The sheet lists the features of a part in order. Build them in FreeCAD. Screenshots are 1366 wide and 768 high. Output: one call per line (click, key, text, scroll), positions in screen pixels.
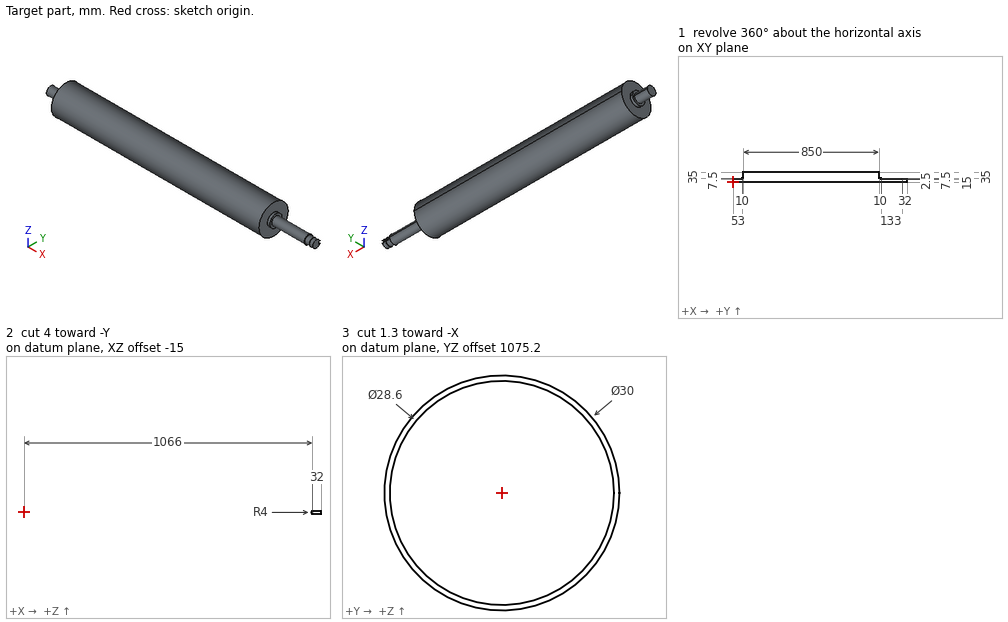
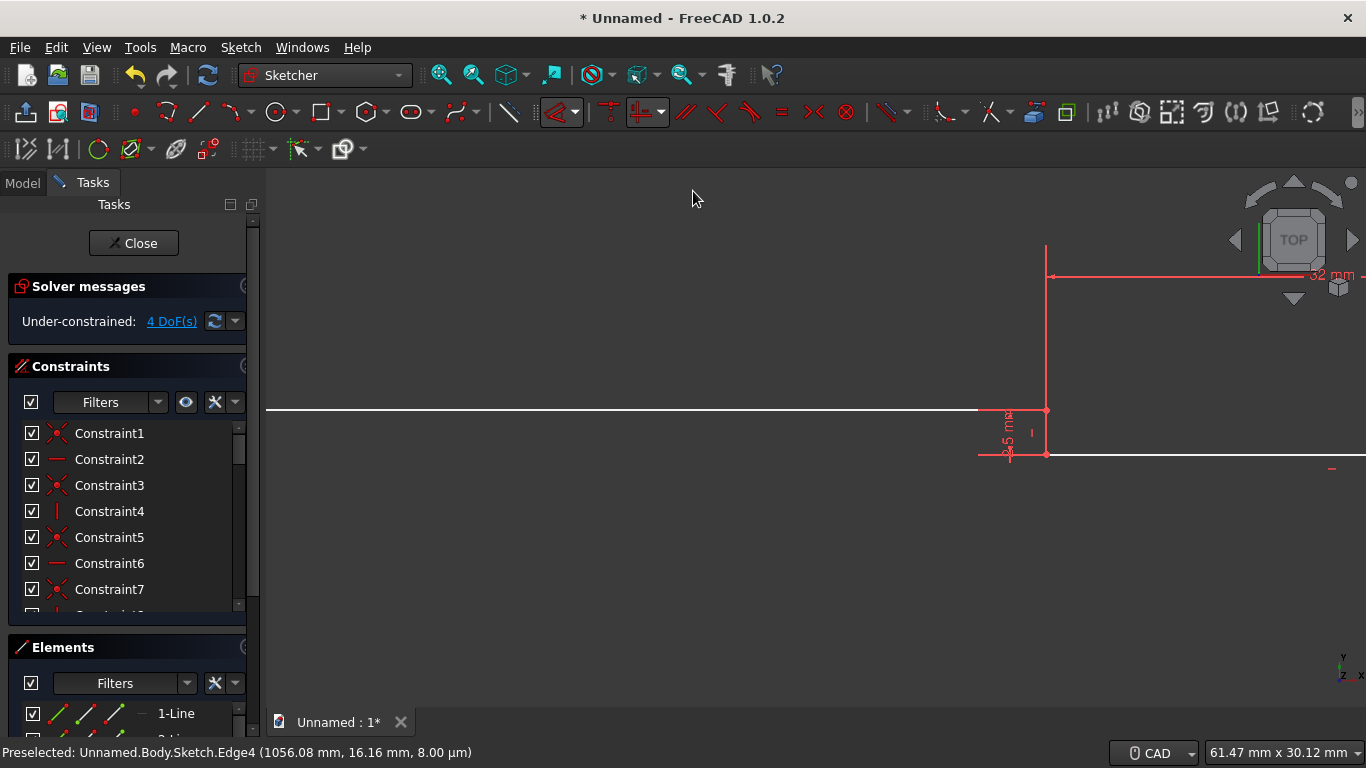
scroll(1124, 448, down, 16)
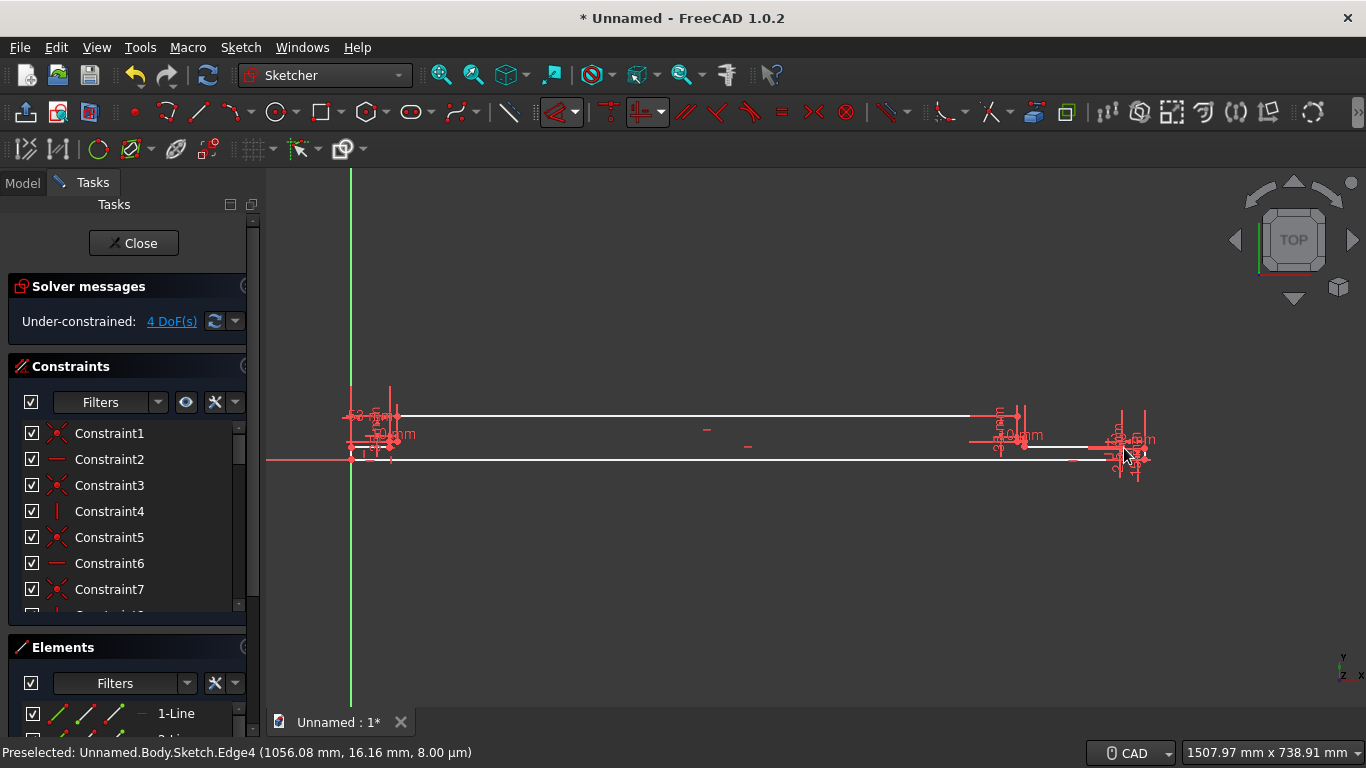
click(1092, 447)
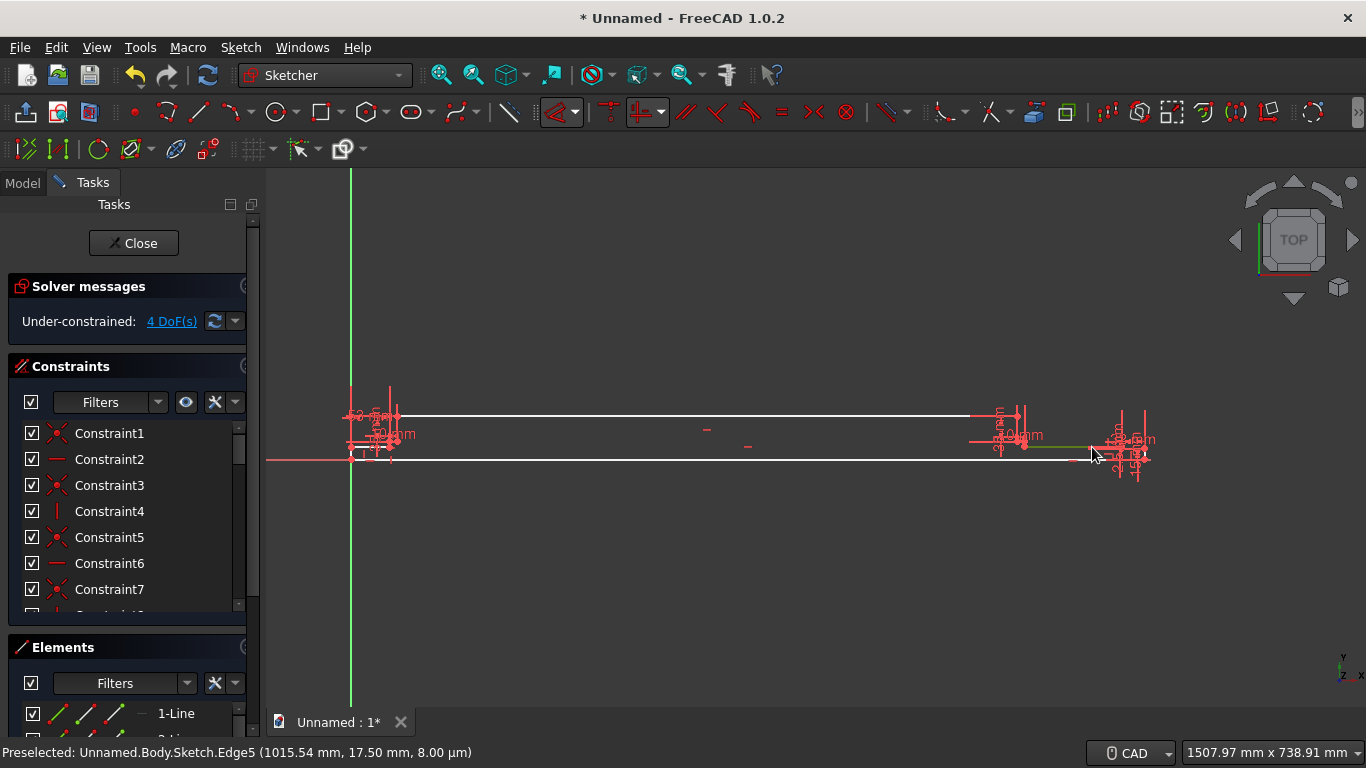
key(l)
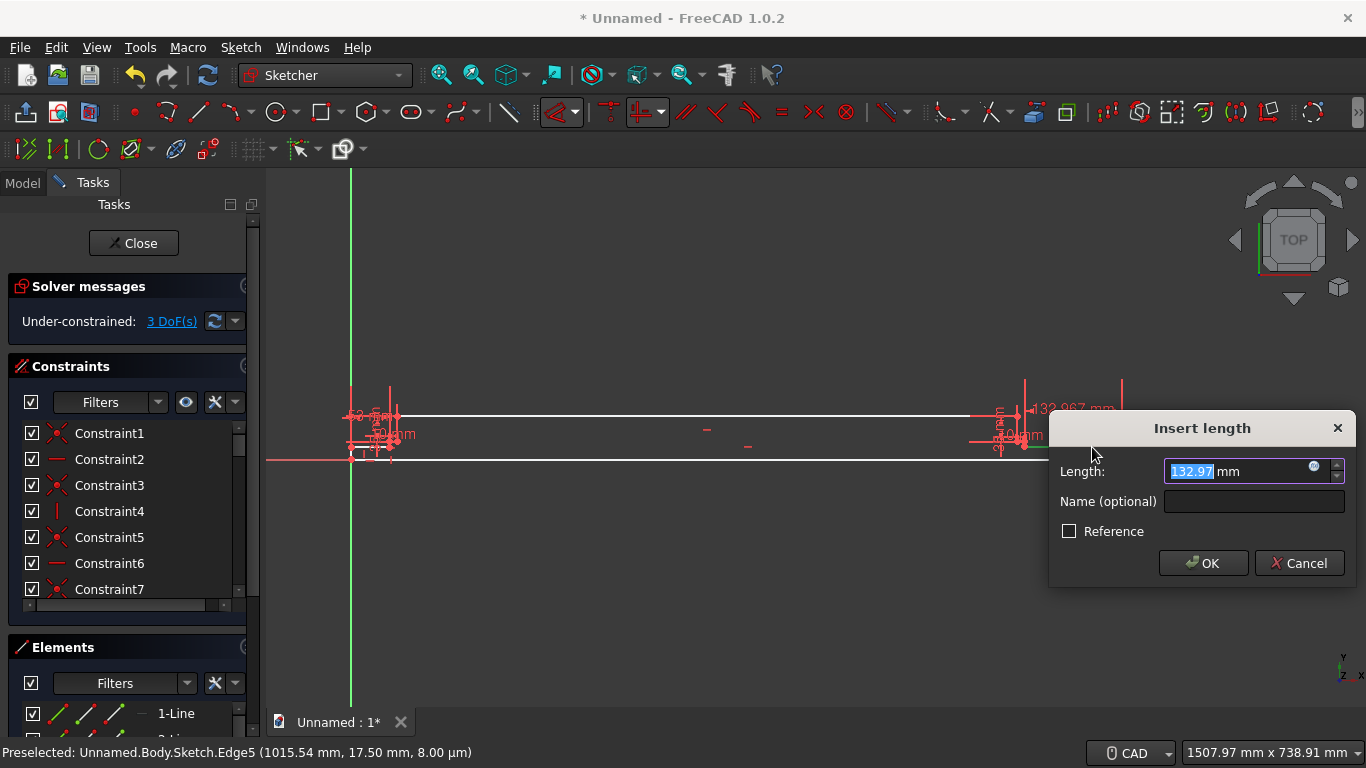
text(133)
key(Return)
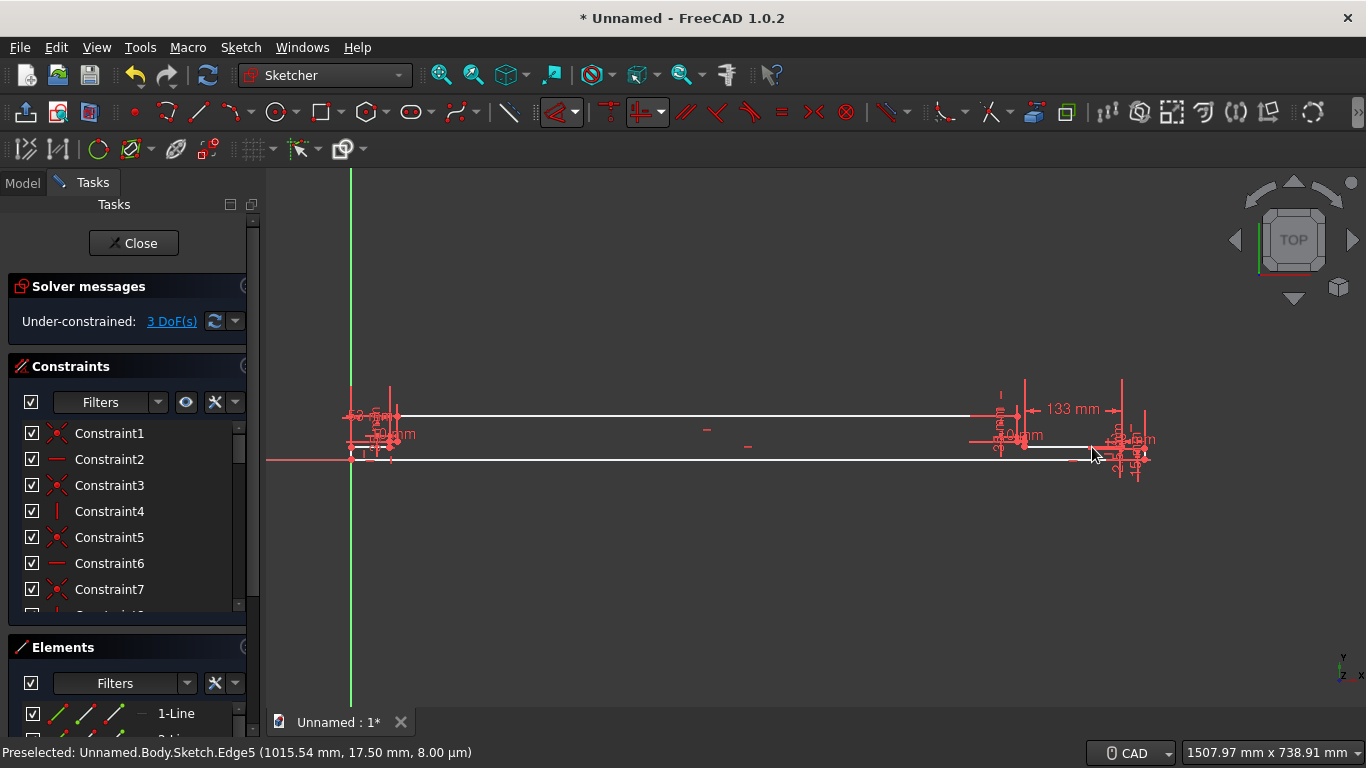
scroll(1025, 444, up, 10)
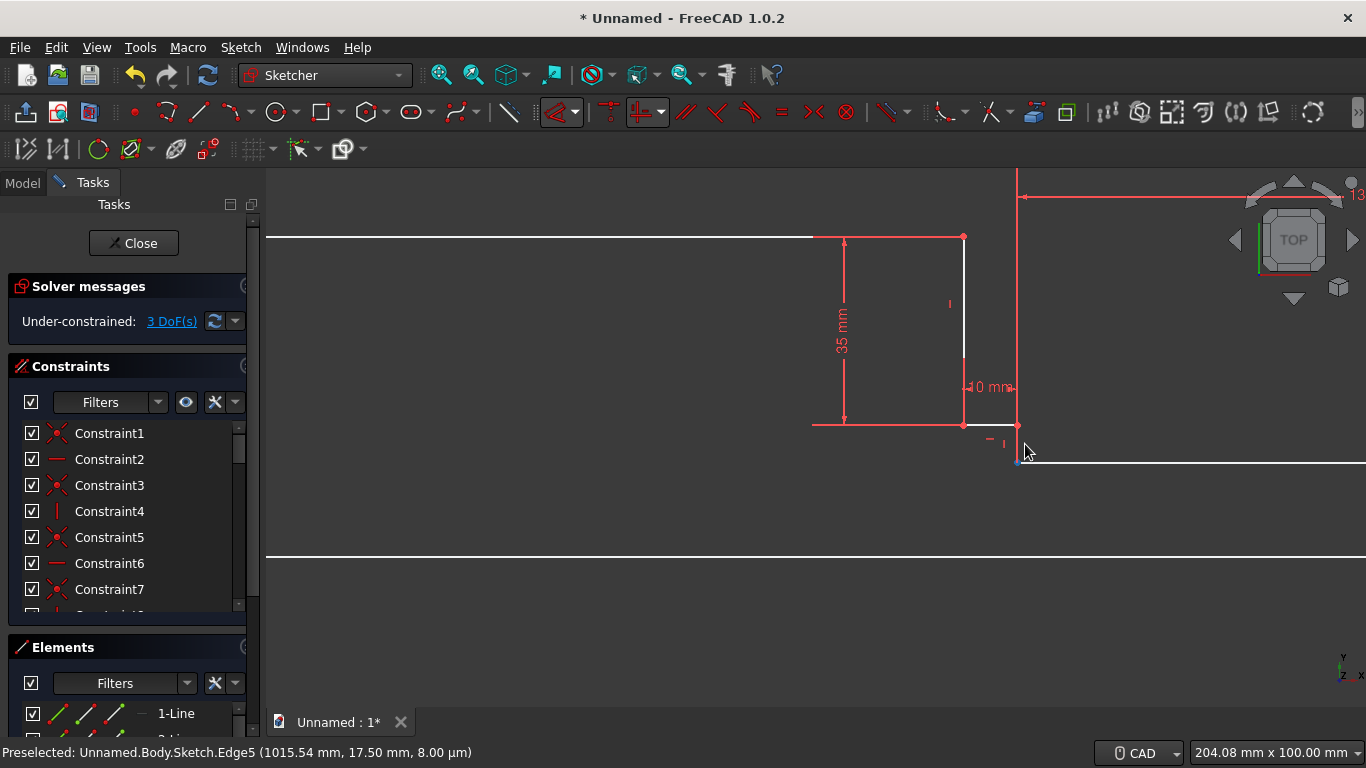
click(1017, 444)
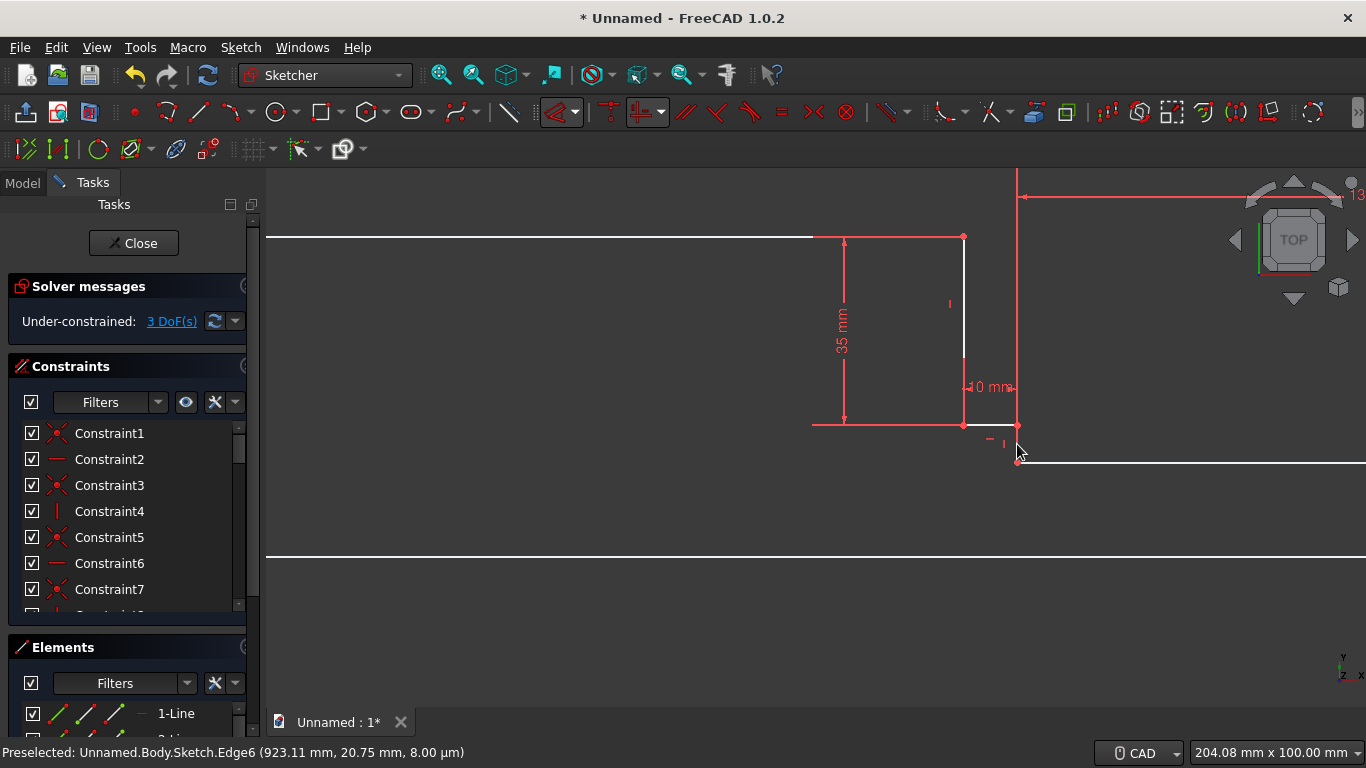
key(i)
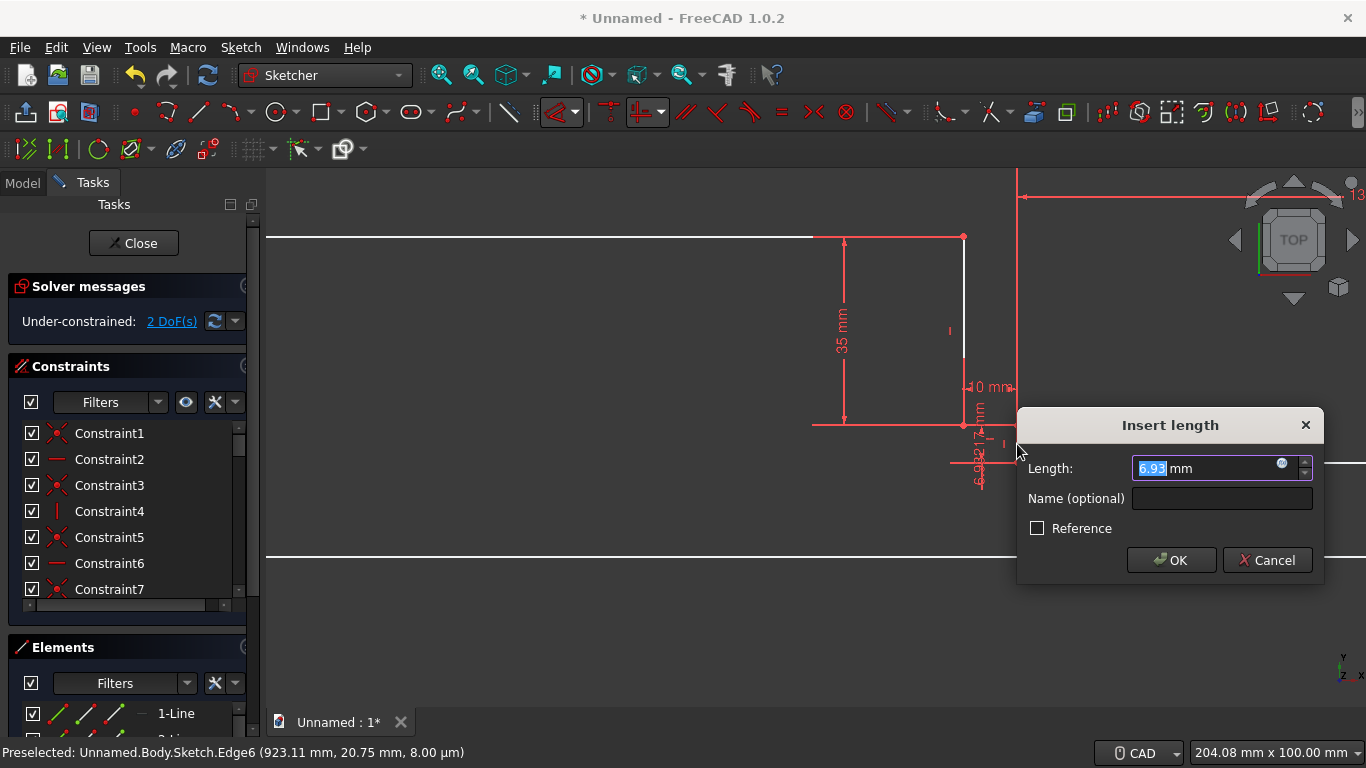
text(7.5)
key(Return)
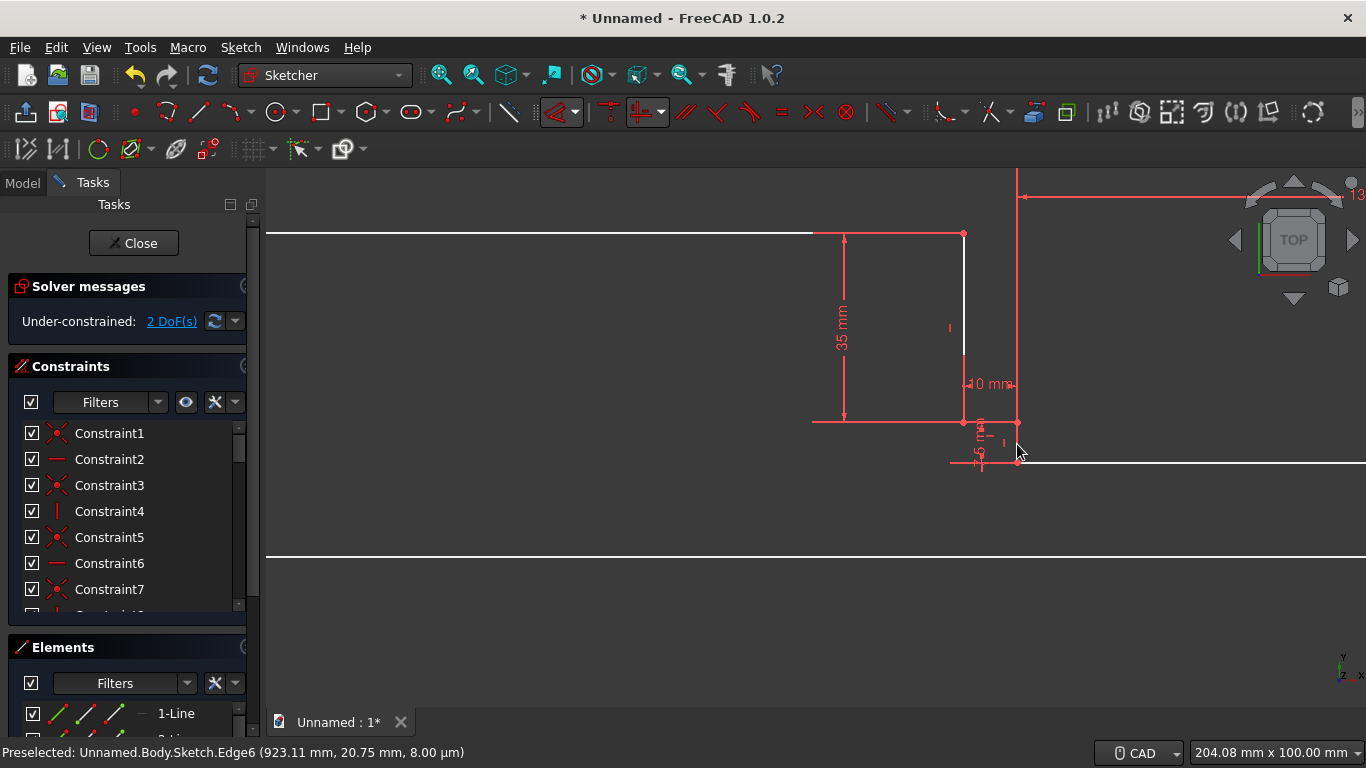
scroll(968, 443, down, 11)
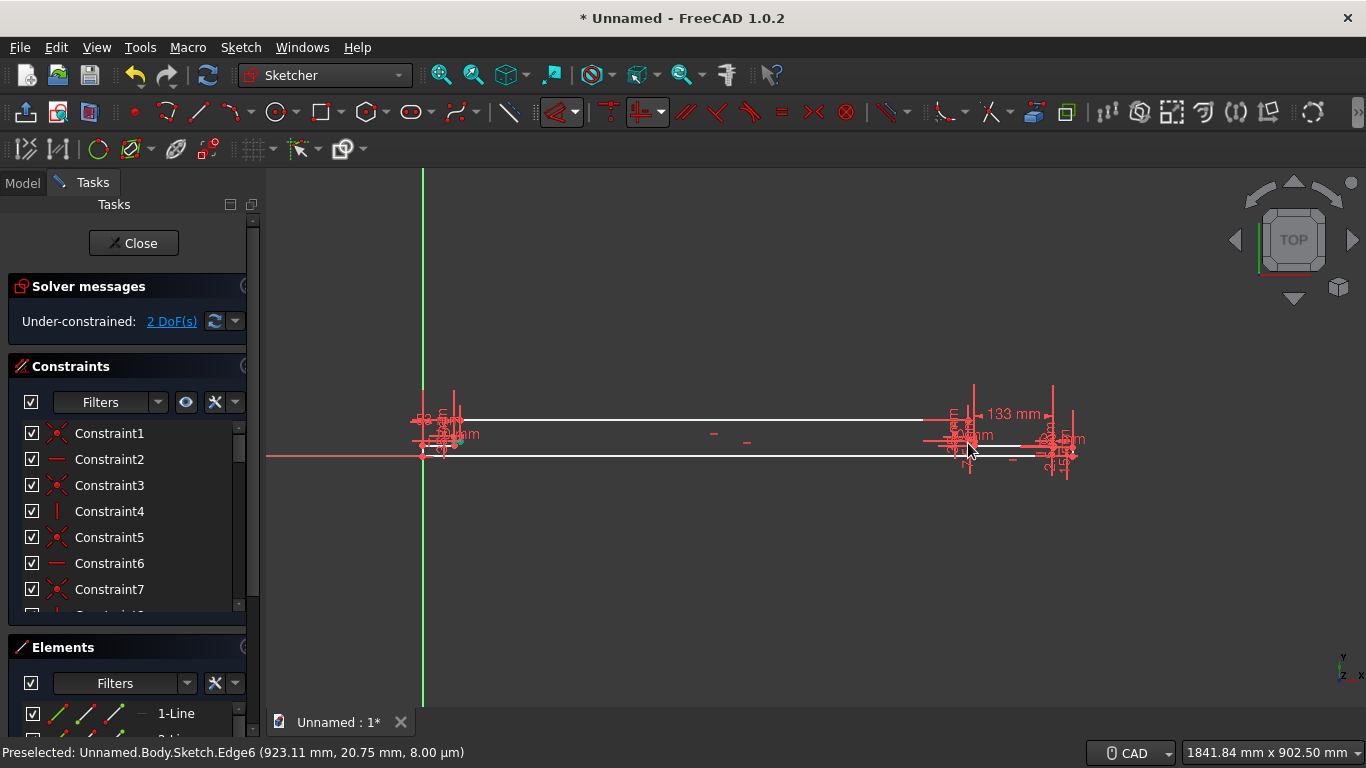
click(816, 420)